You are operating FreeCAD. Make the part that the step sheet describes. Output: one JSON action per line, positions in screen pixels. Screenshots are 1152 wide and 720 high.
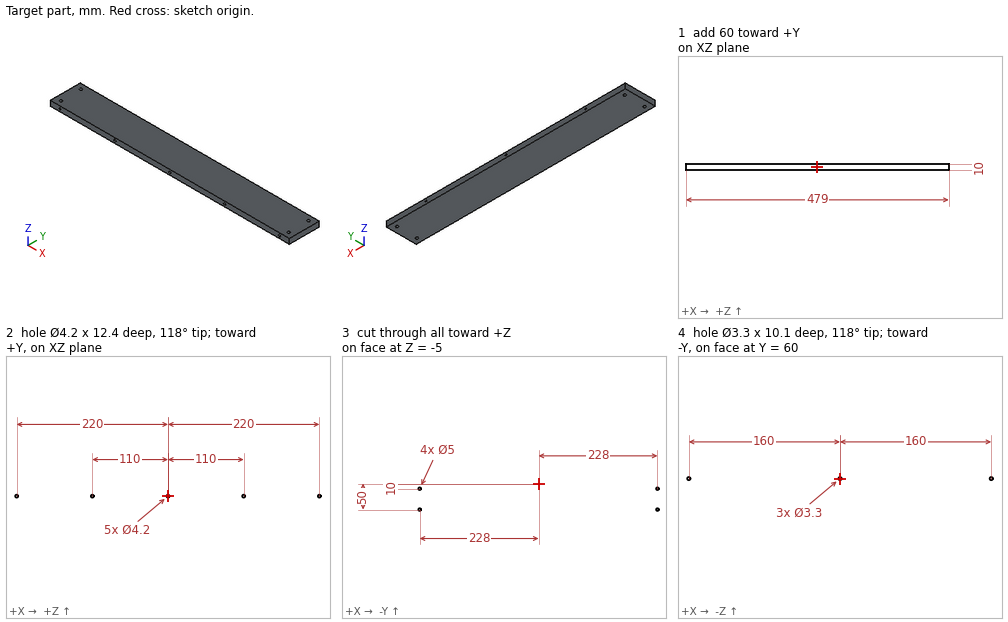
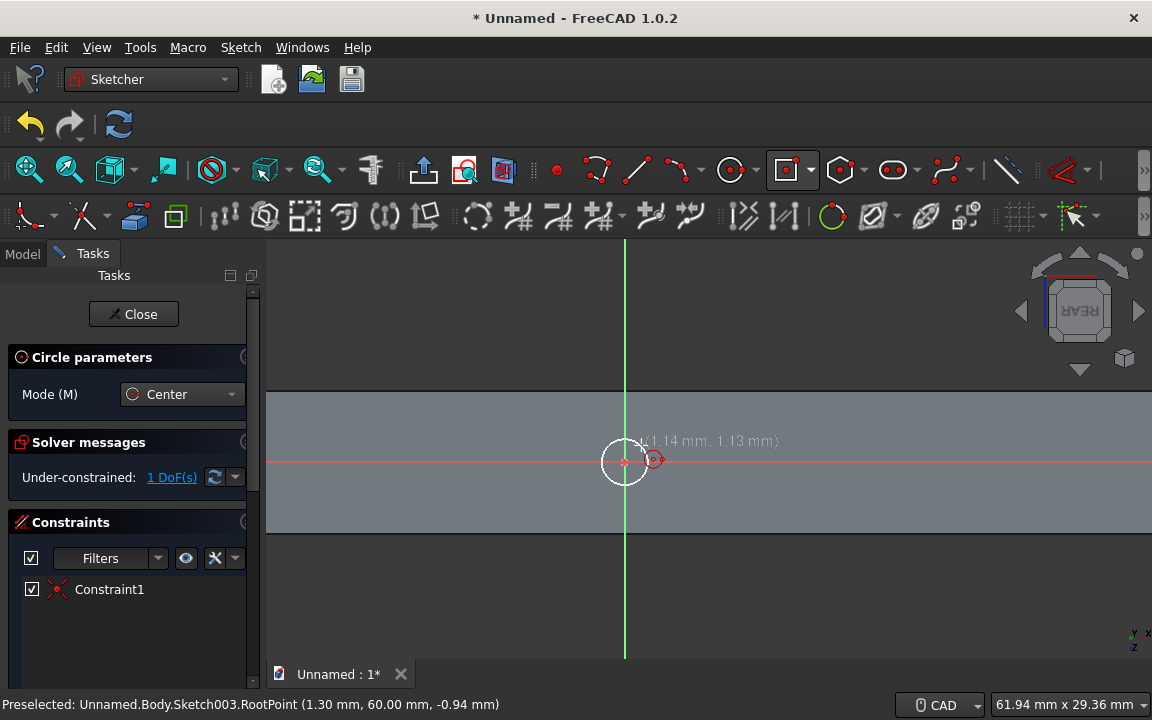
{"action": "scroll", "coordinate": [642, 447], "scroll_direction": "down", "scroll_amount": 11}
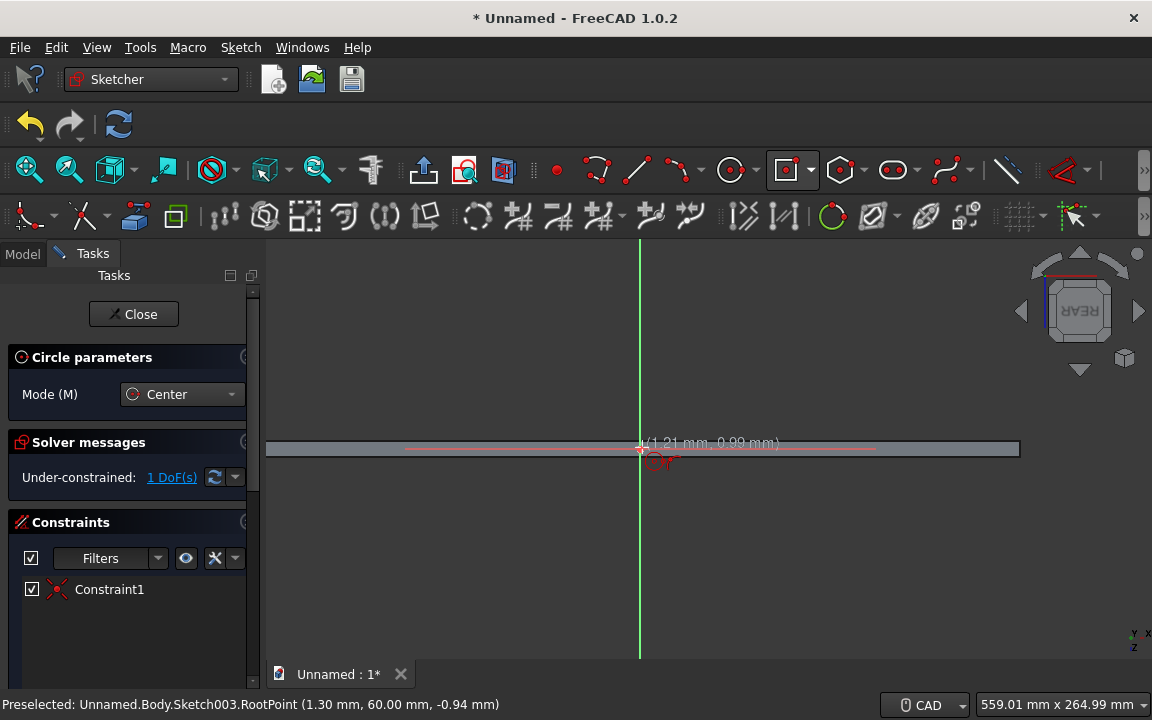
{"action": "scroll", "coordinate": [387, 449], "scroll_direction": "up", "scroll_amount": 11}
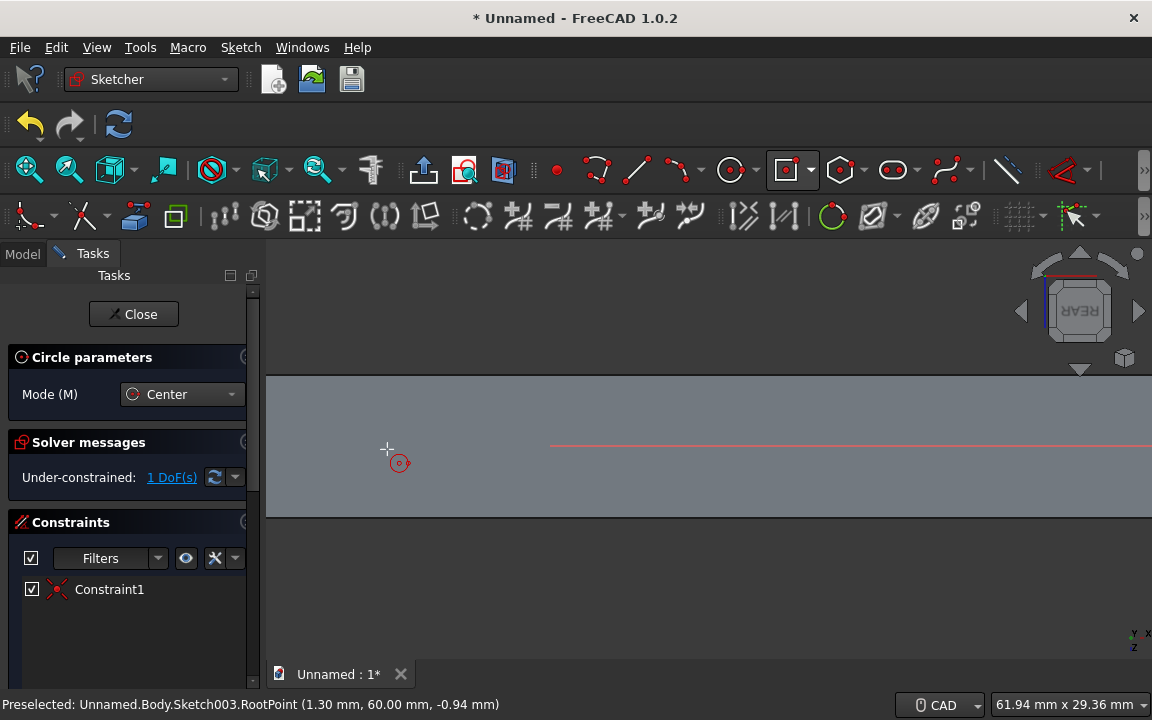
{"action": "scroll", "coordinate": [387, 449], "scroll_direction": "down", "scroll_amount": 11}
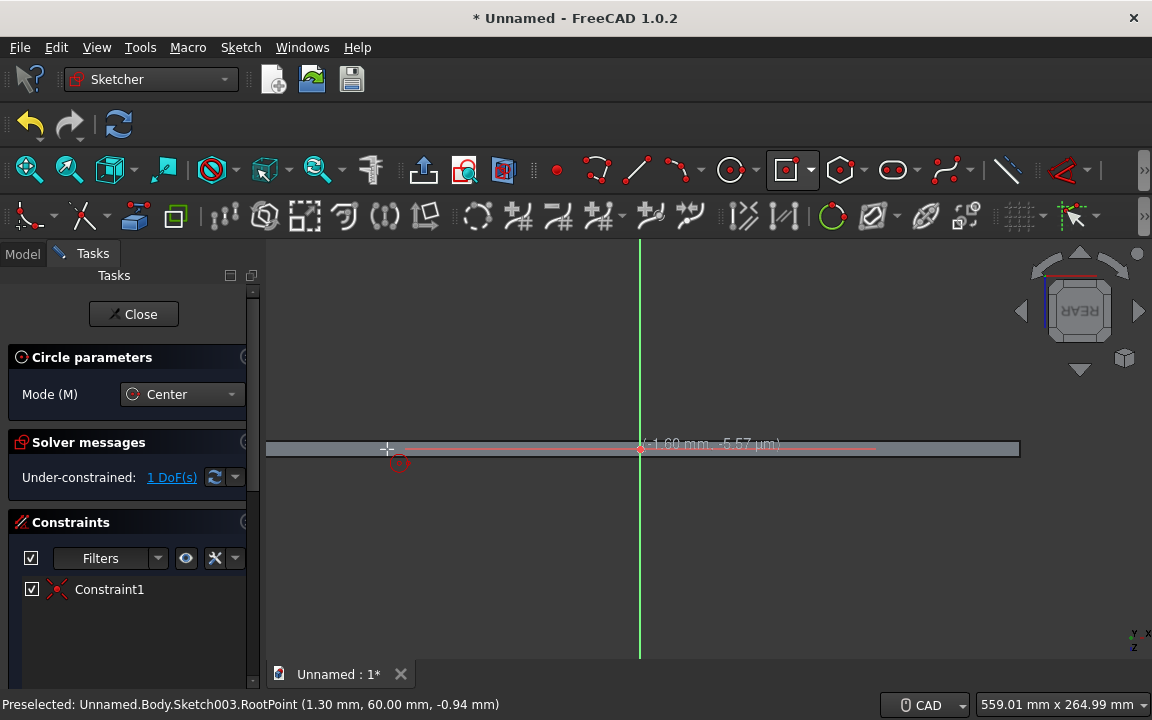
{"action": "left_click", "coordinate": [387, 449]}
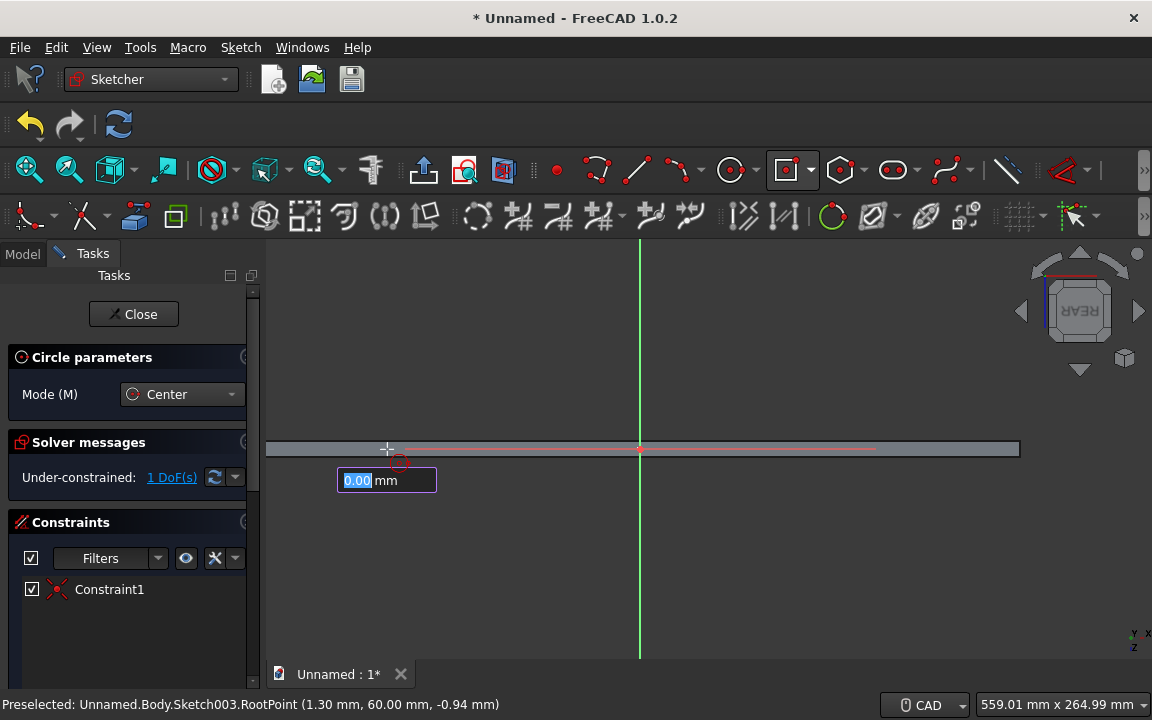
{"action": "scroll", "coordinate": [386, 452], "scroll_direction": "up", "scroll_amount": 10}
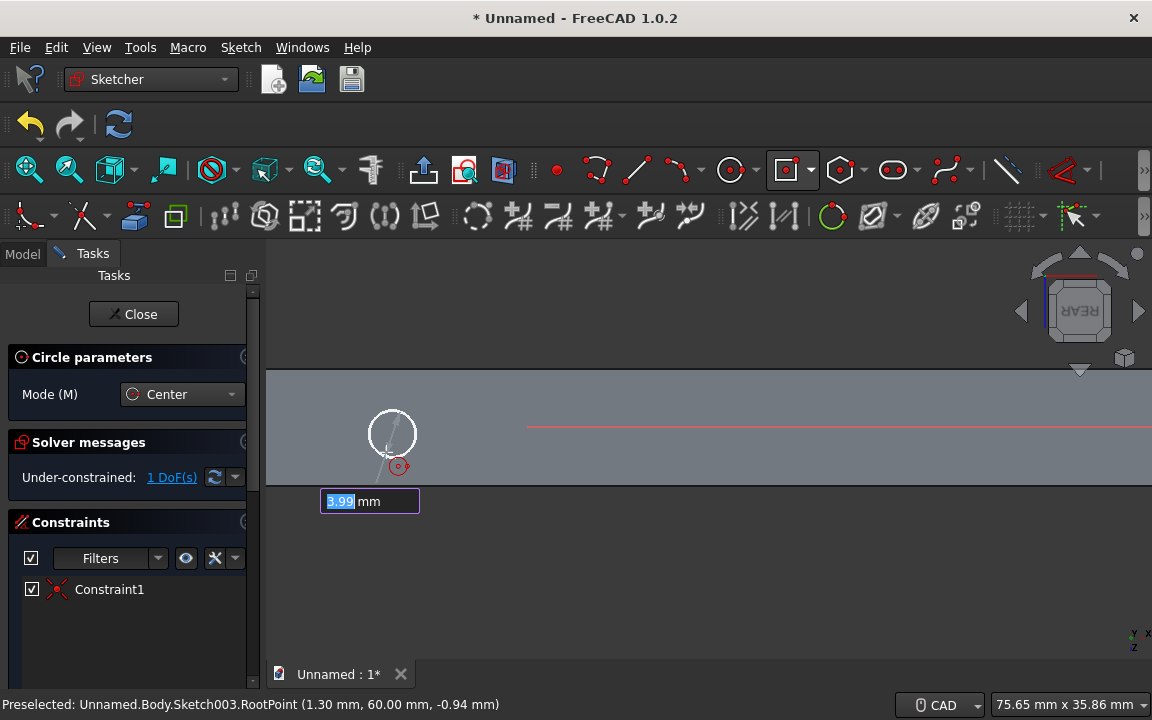
{"action": "left_click", "coordinate": [385, 446]}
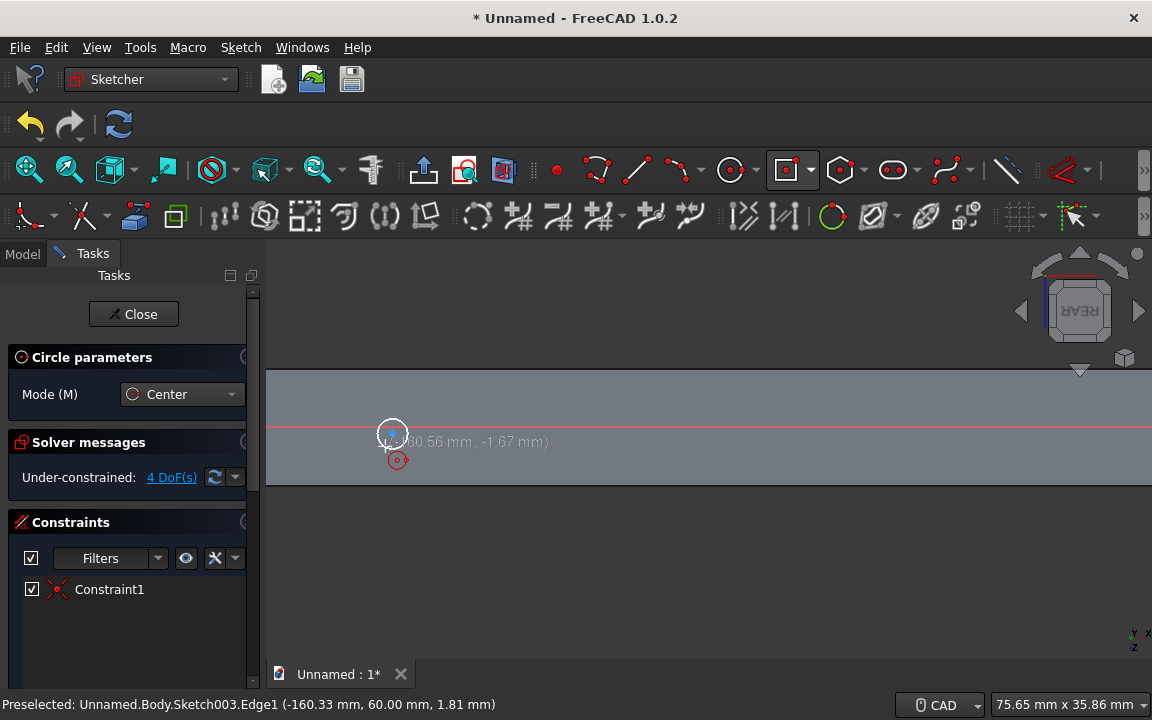
{"action": "scroll", "coordinate": [386, 452], "scroll_direction": "down", "scroll_amount": 10}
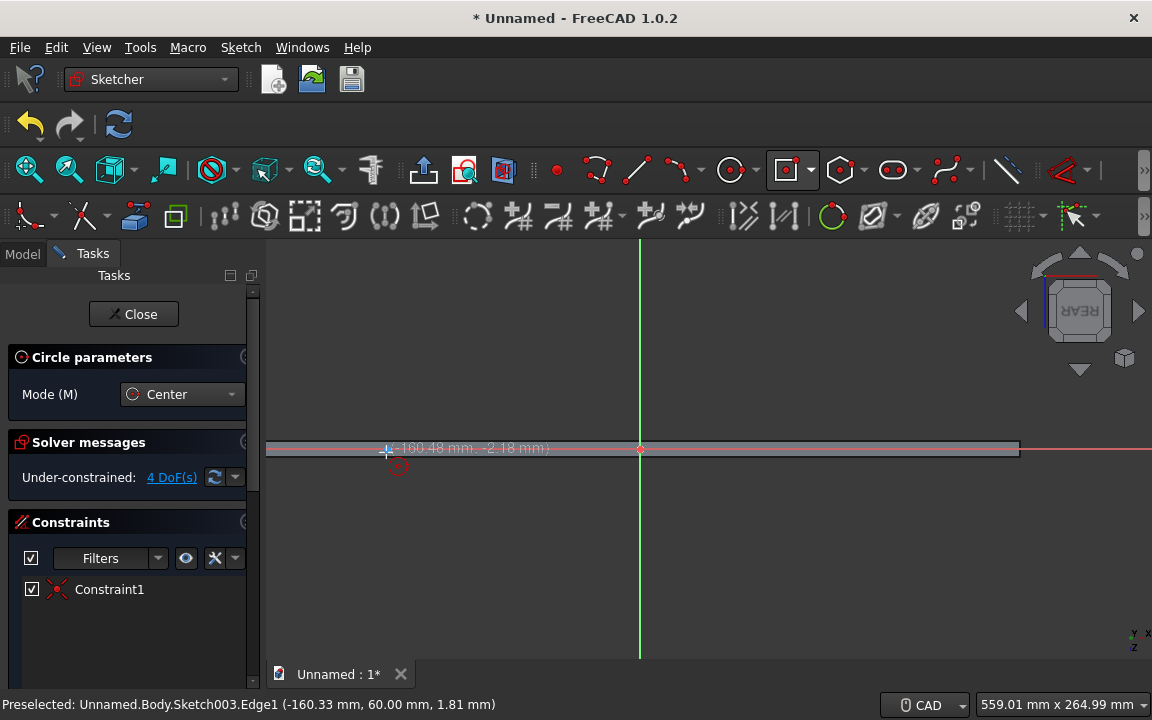
{"action": "scroll", "coordinate": [894, 449], "scroll_direction": "up", "scroll_amount": 11}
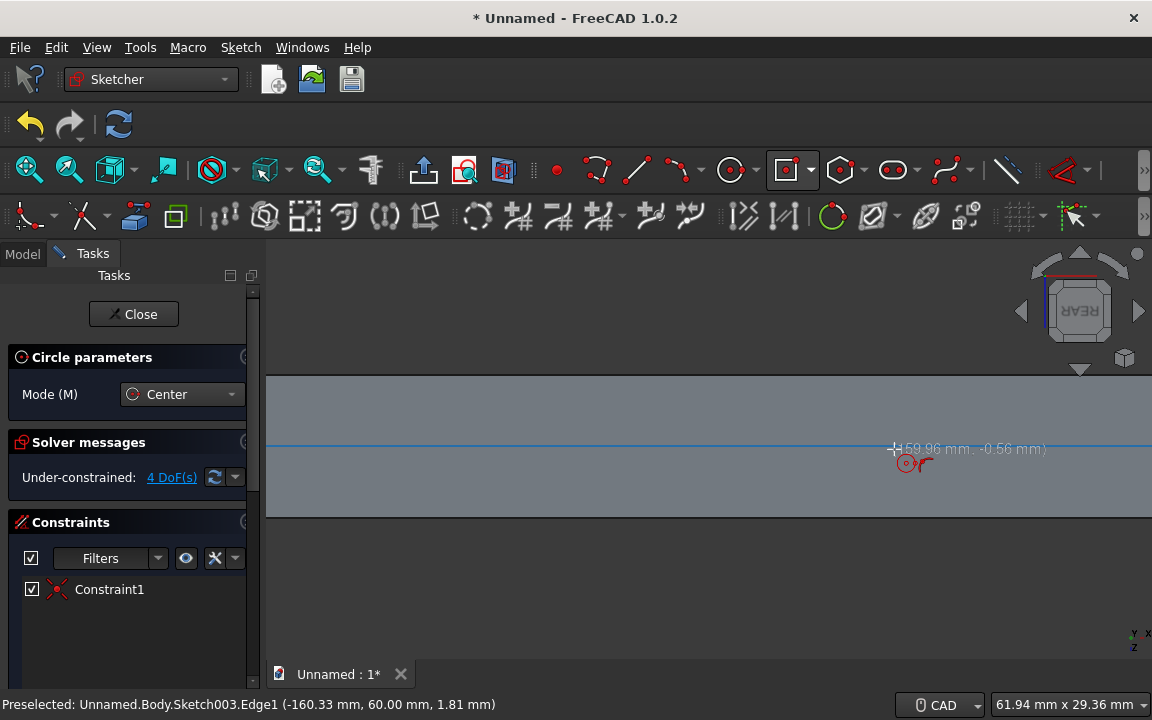
{"action": "scroll", "coordinate": [895, 449], "scroll_direction": "down", "scroll_amount": 11}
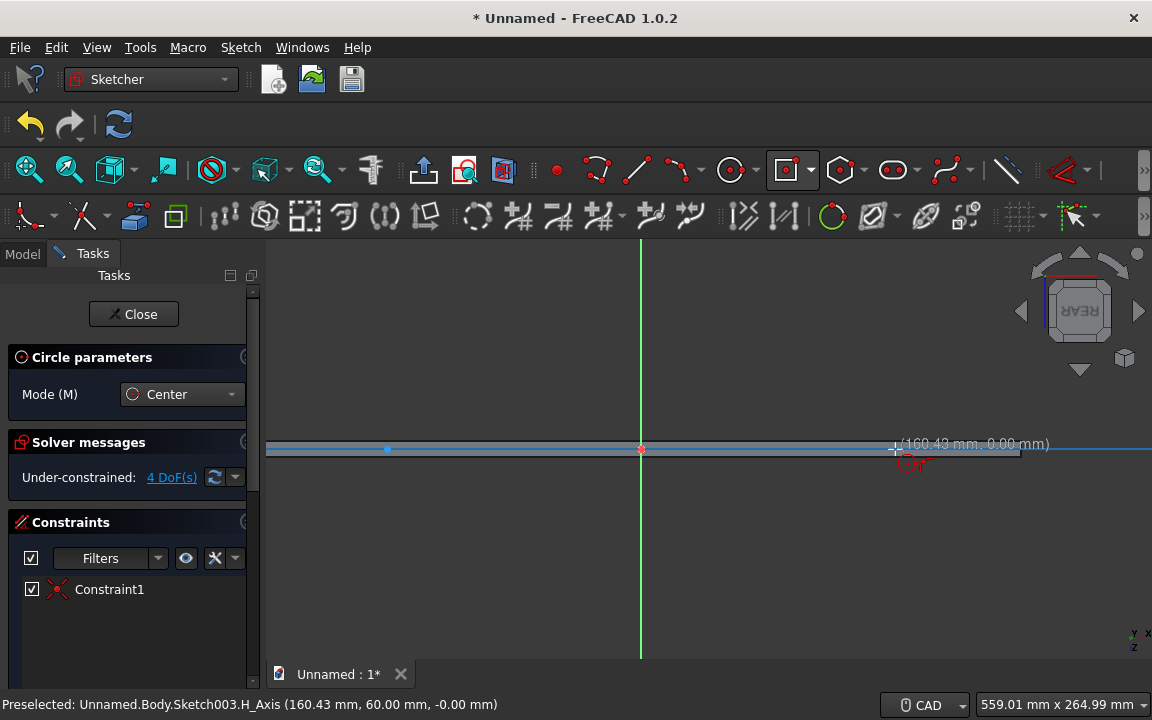
{"action": "left_click", "coordinate": [895, 449]}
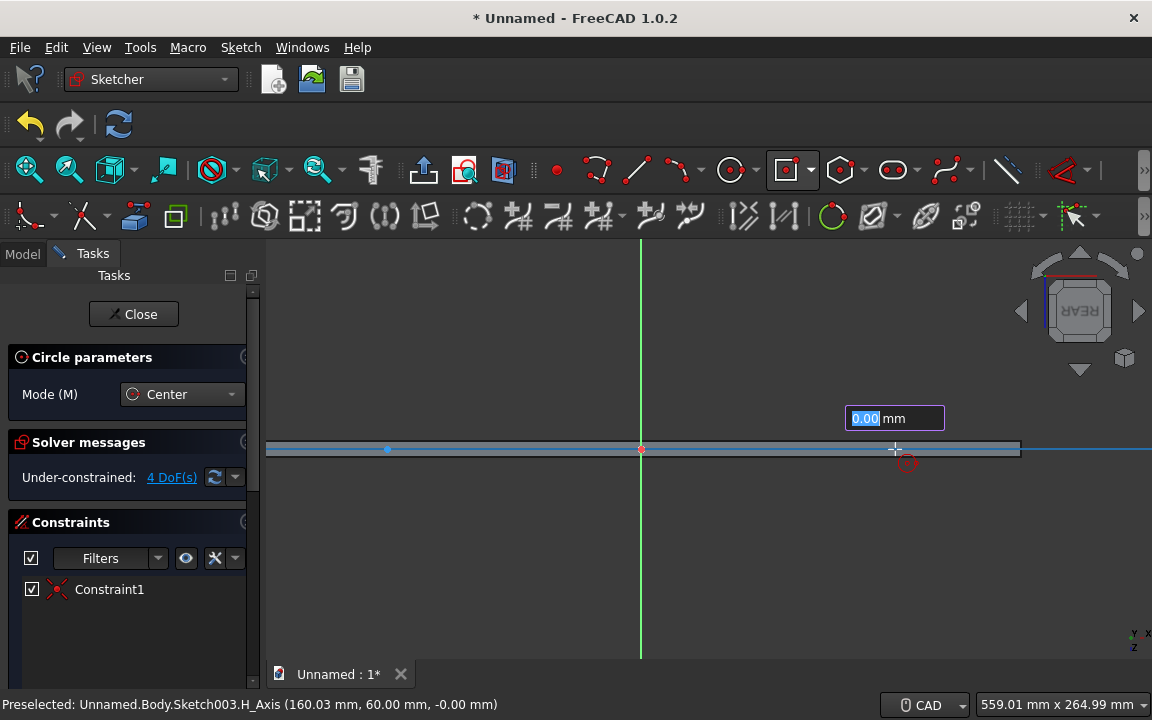
{"action": "scroll", "coordinate": [896, 447], "scroll_direction": "up", "scroll_amount": 10}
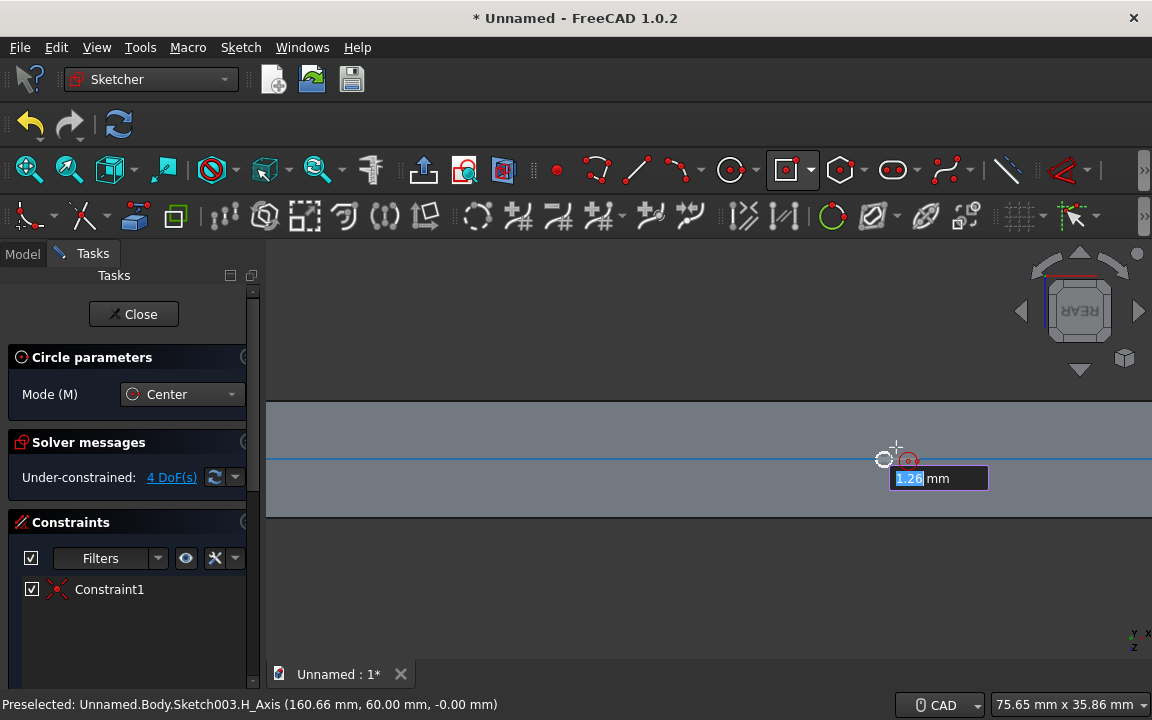
{"action": "left_click", "coordinate": [890, 441]}
{"action": "key", "text": "Escape"}